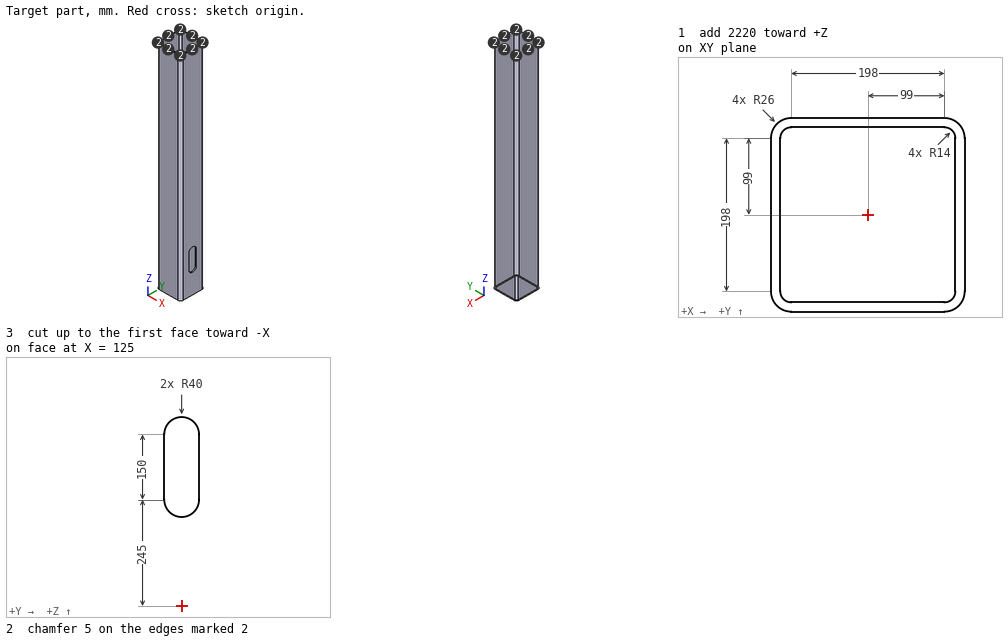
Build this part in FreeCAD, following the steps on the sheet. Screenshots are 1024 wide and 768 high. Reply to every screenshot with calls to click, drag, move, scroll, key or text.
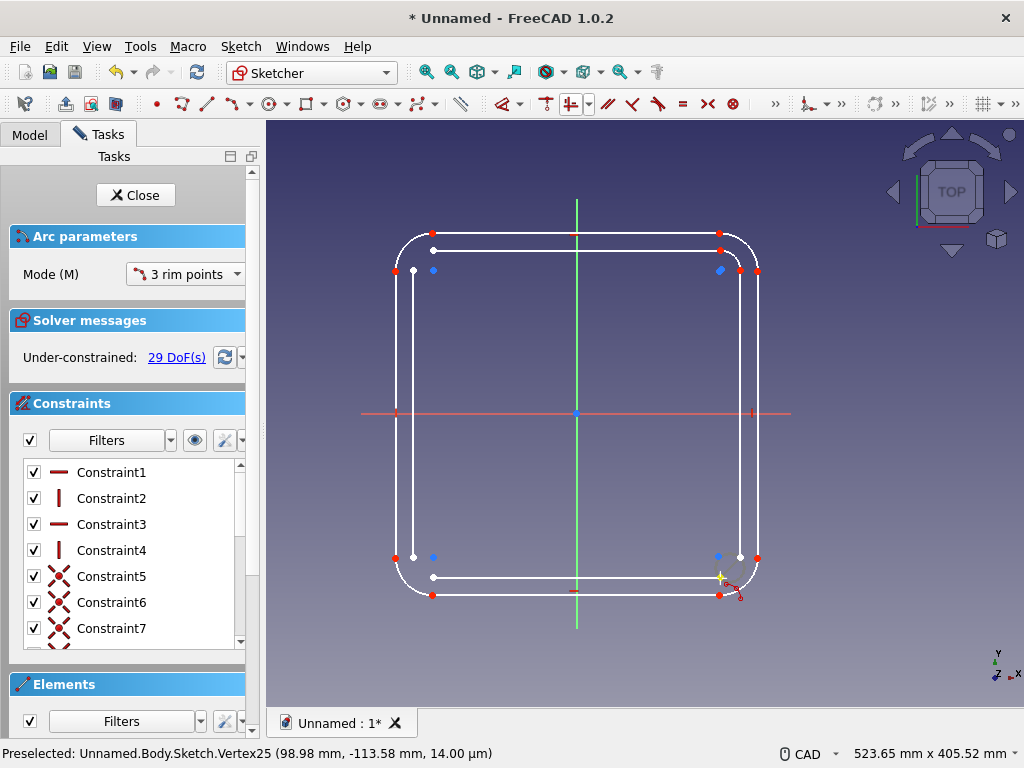
scroll(734, 571, up, 5)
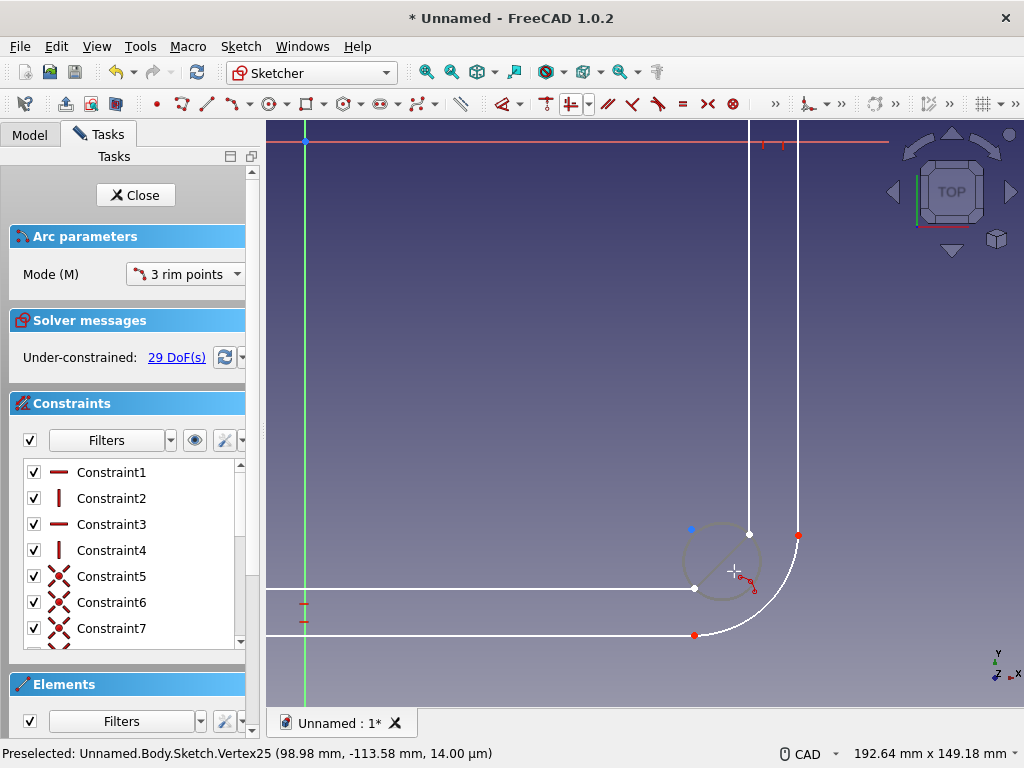
click(734, 570)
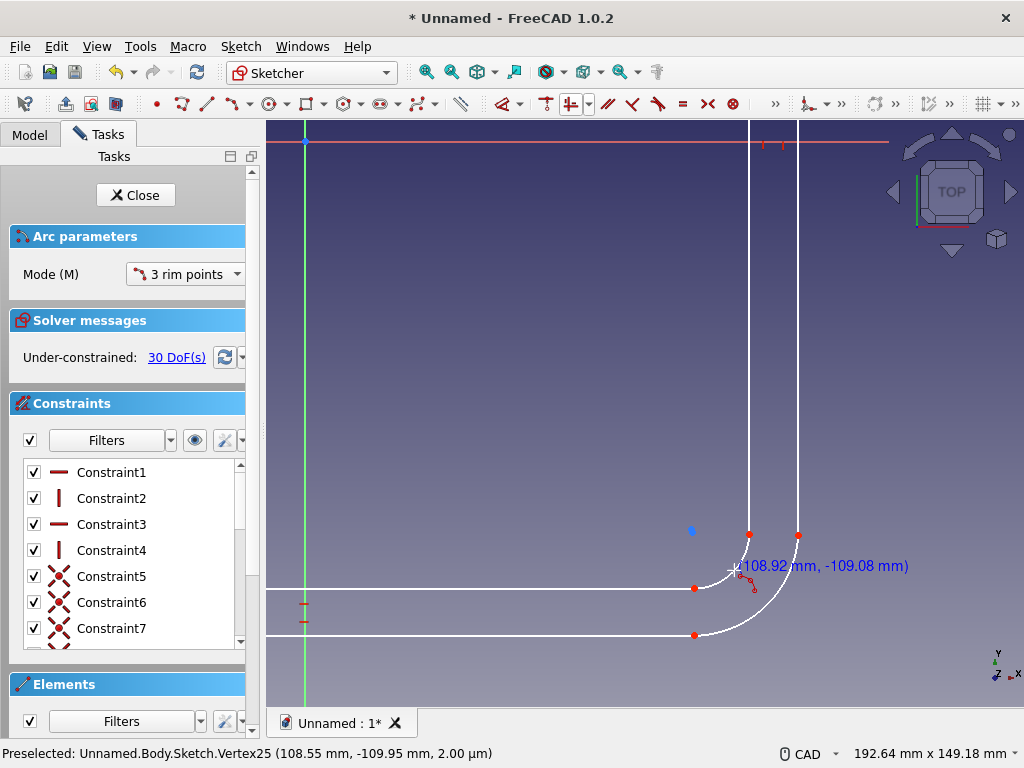
scroll(734, 572, down, 5)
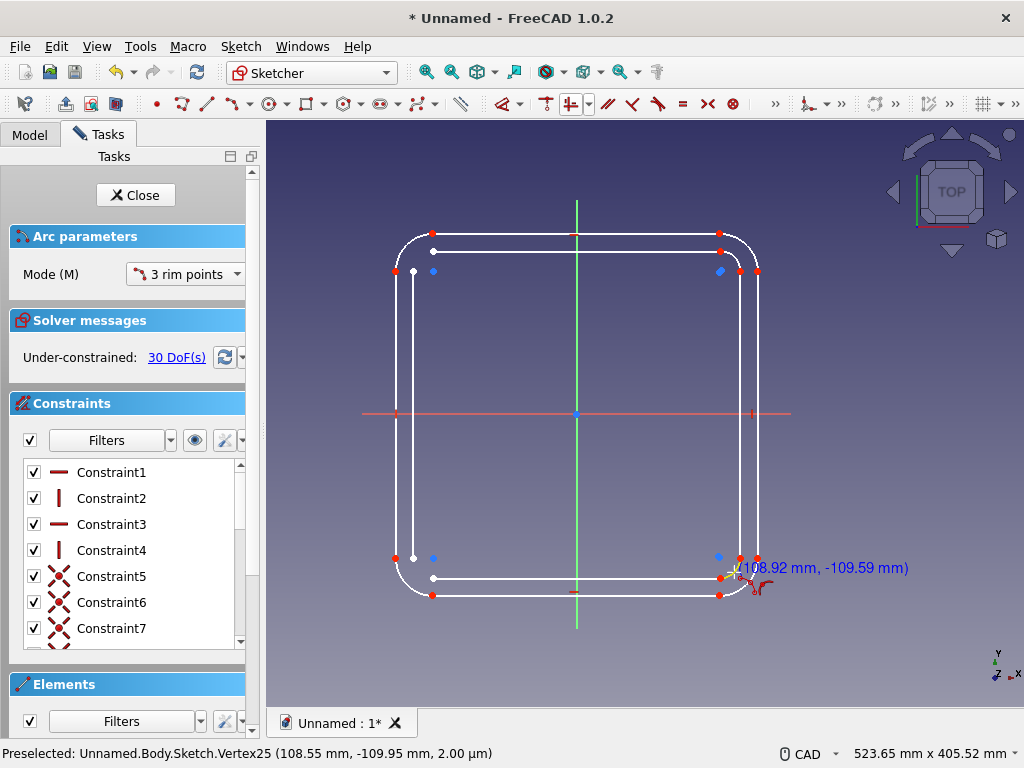
click(433, 579)
click(413, 559)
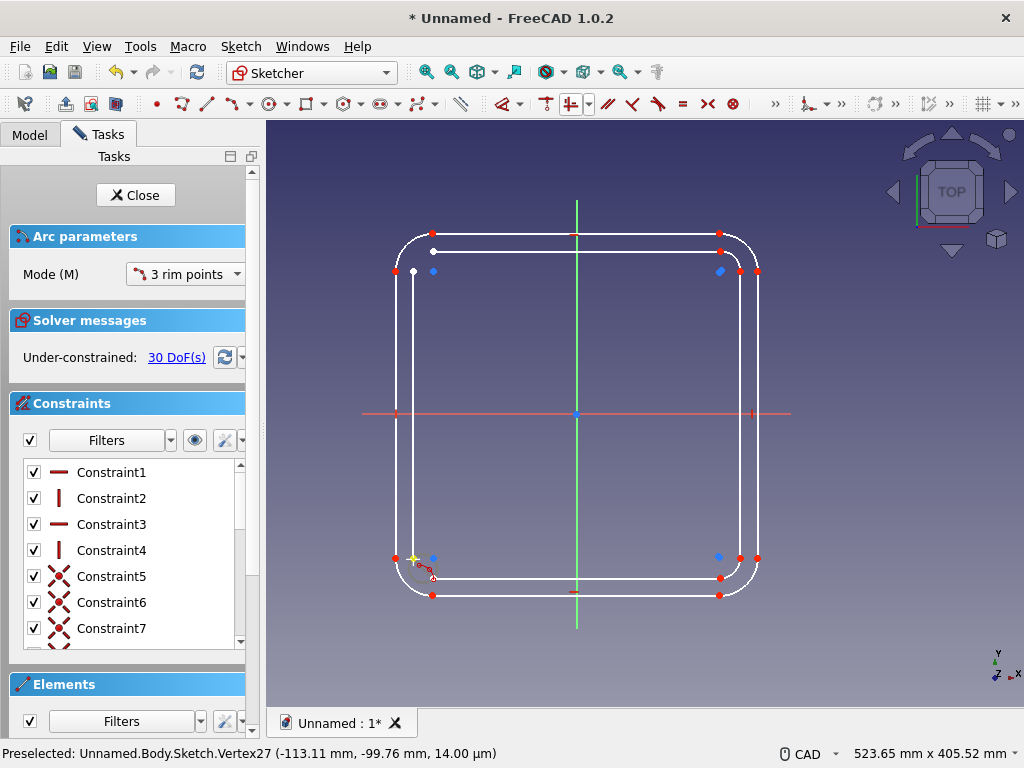
scroll(419, 572, up, 5)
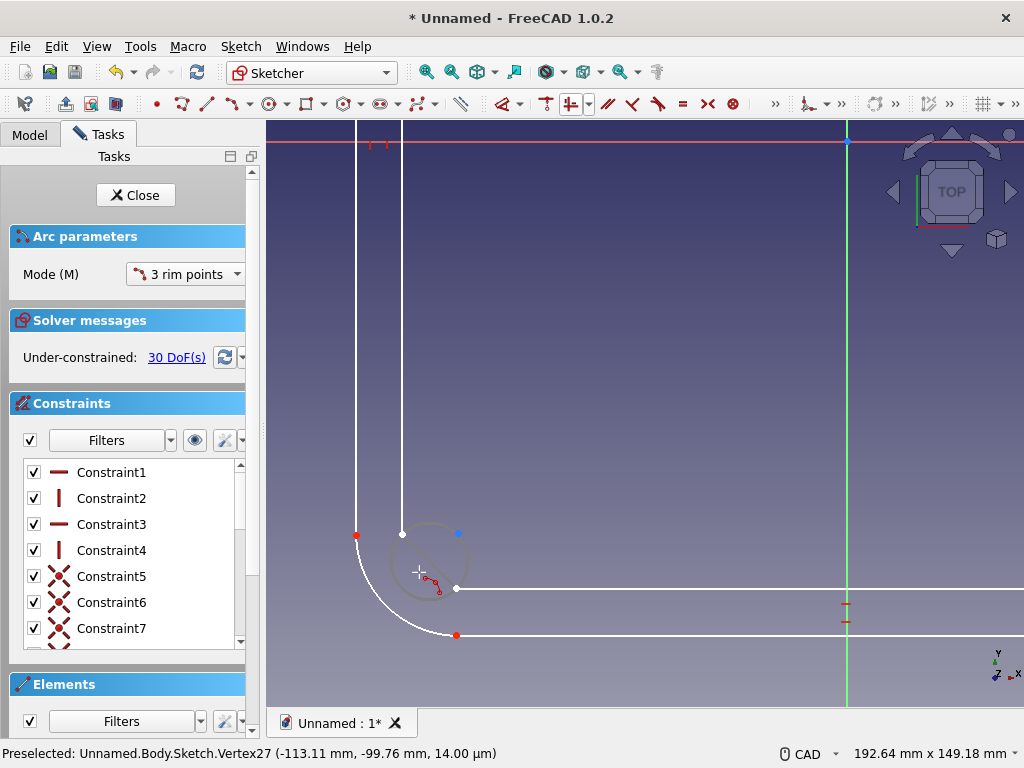
click(419, 570)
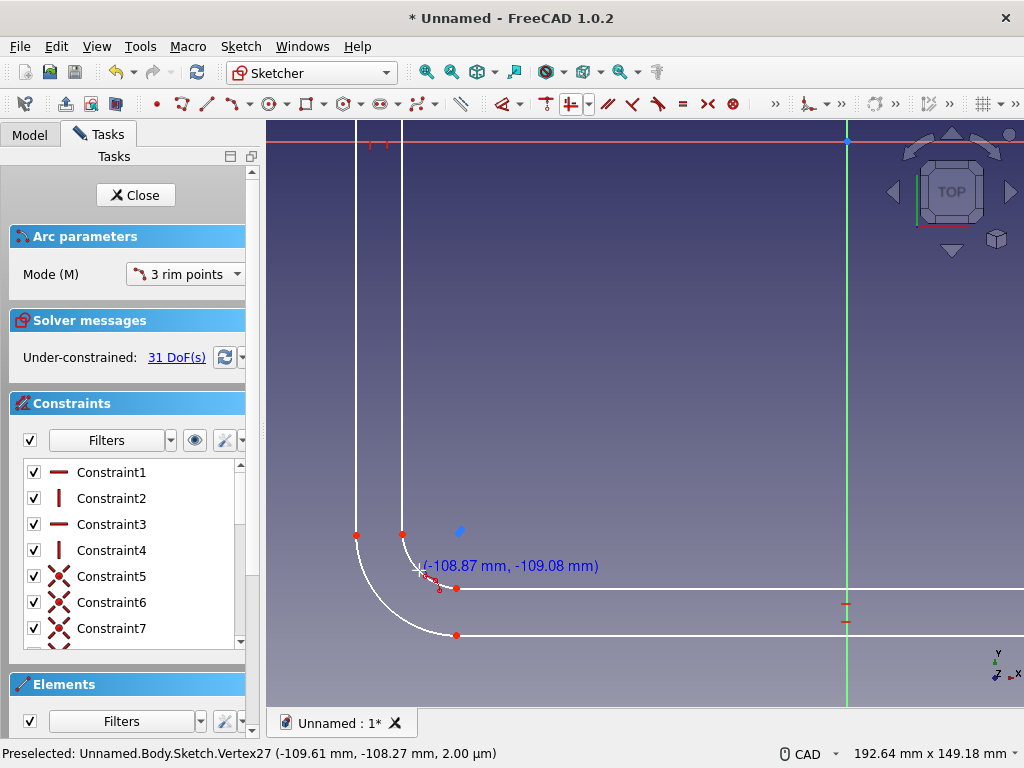
scroll(419, 572, down, 5)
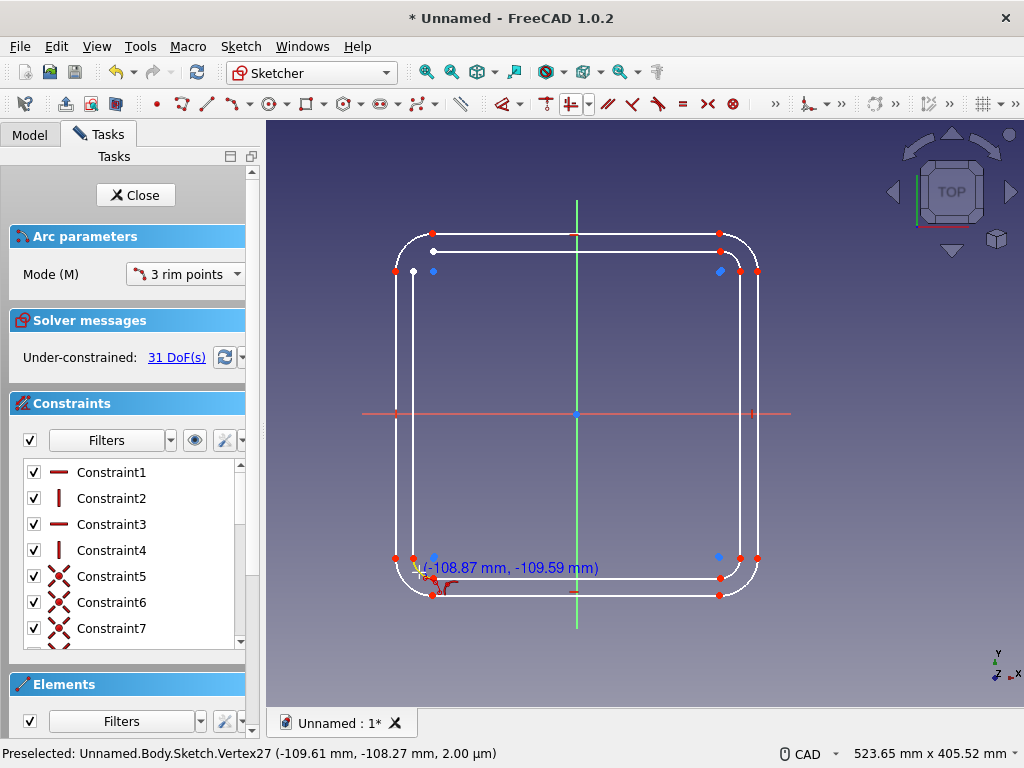
click(413, 272)
click(433, 252)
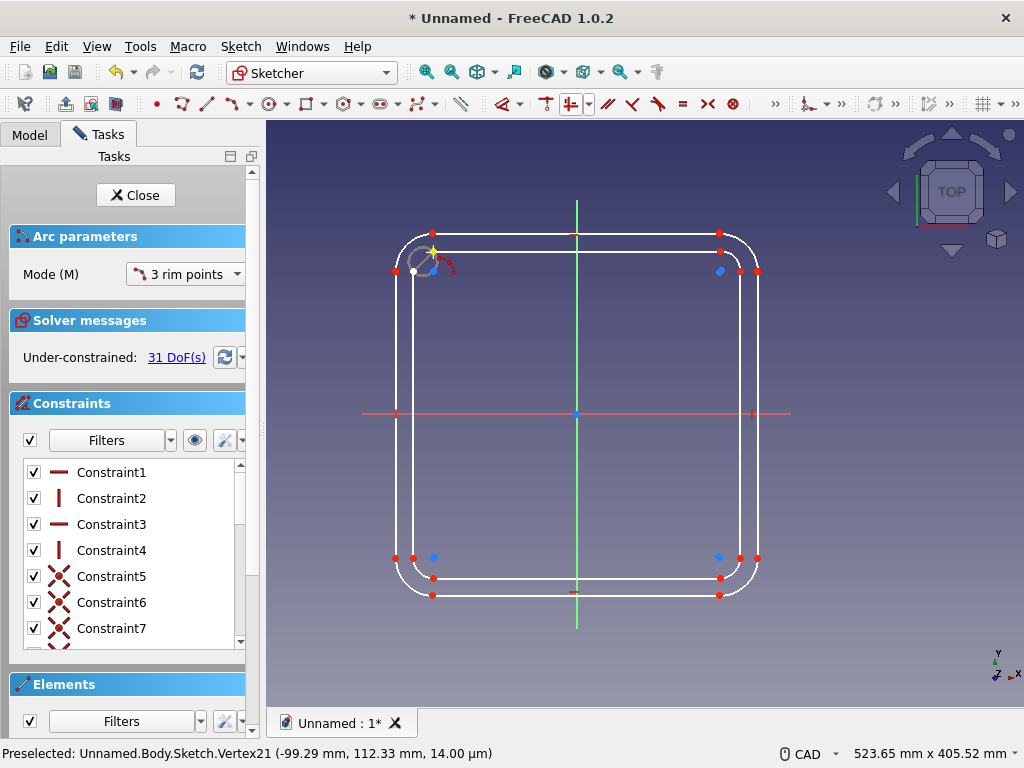
scroll(419, 257, up, 5)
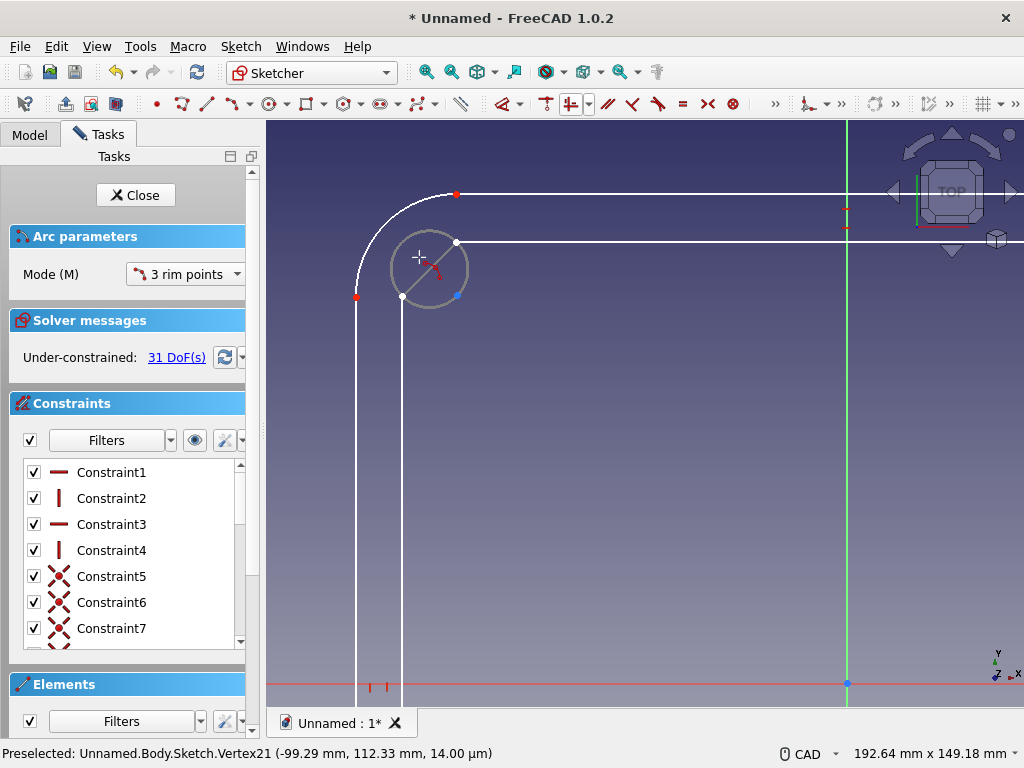
click(419, 255)
key(Escape)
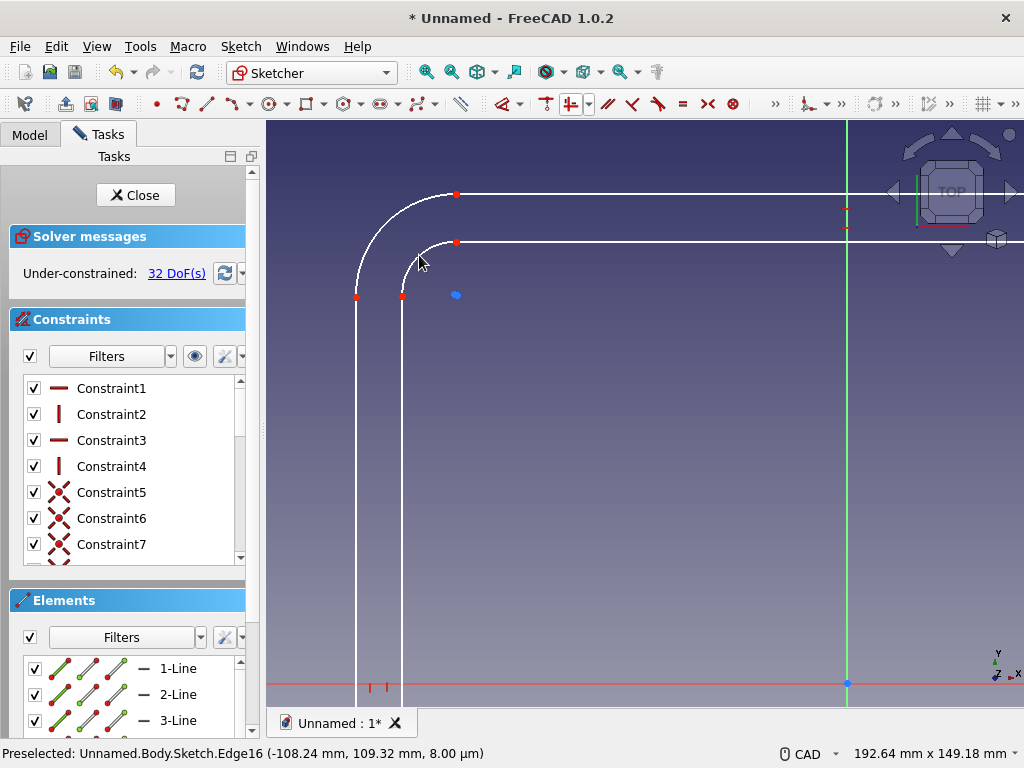
click(691, 194)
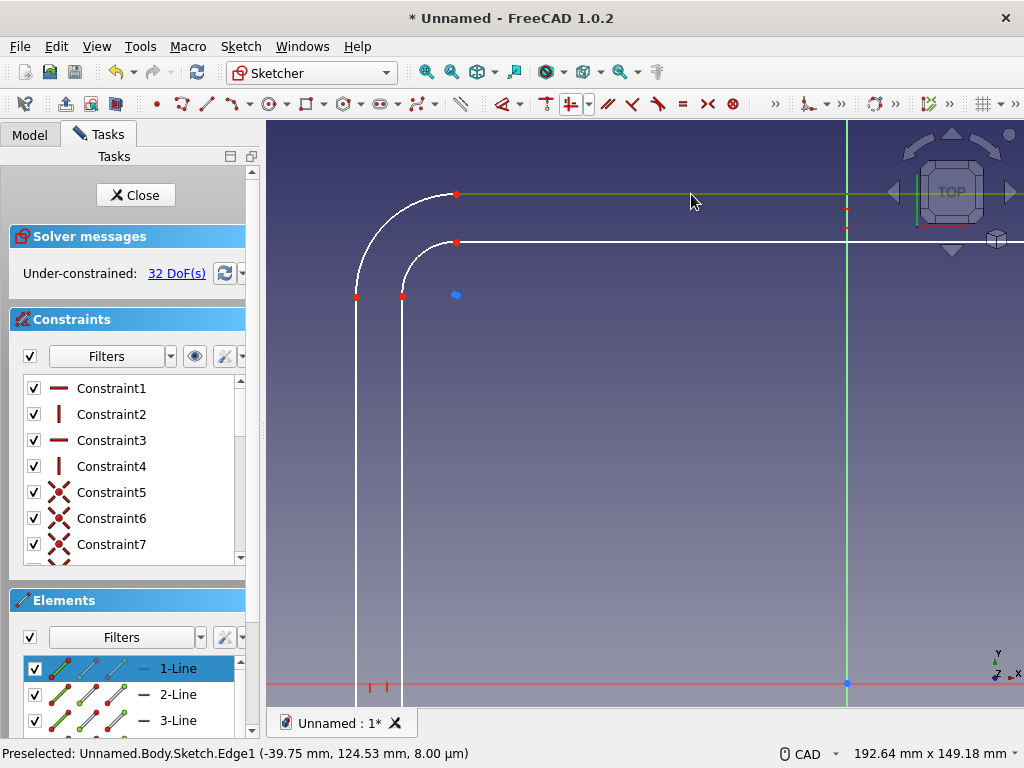
click(410, 206)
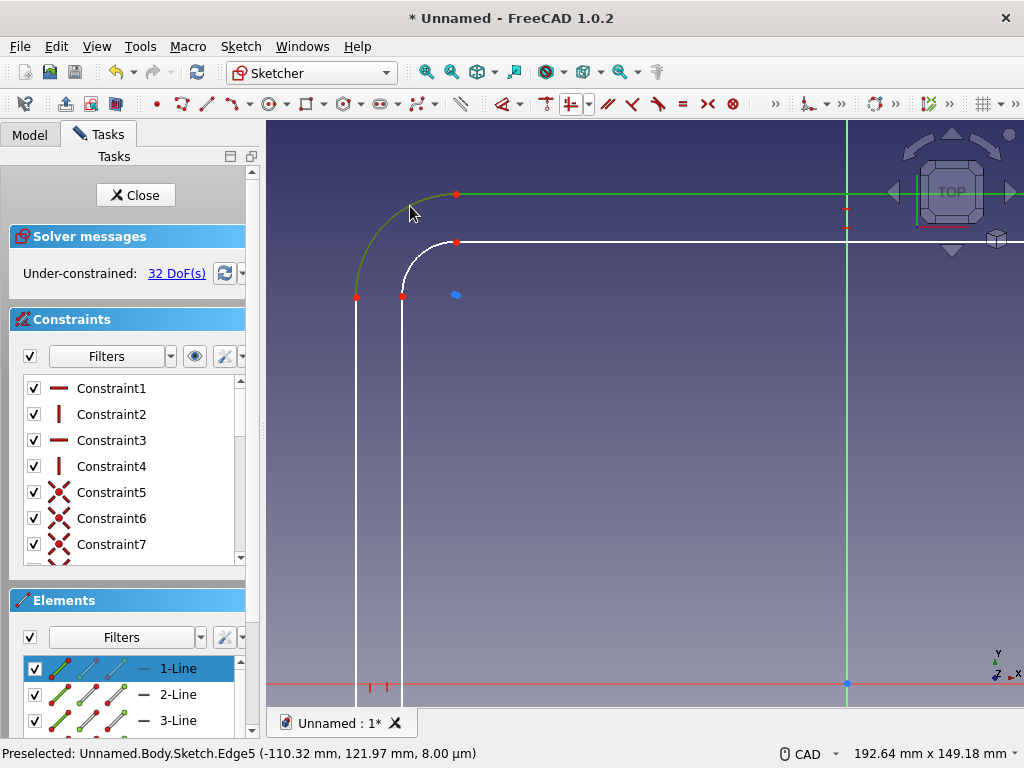
click(658, 104)